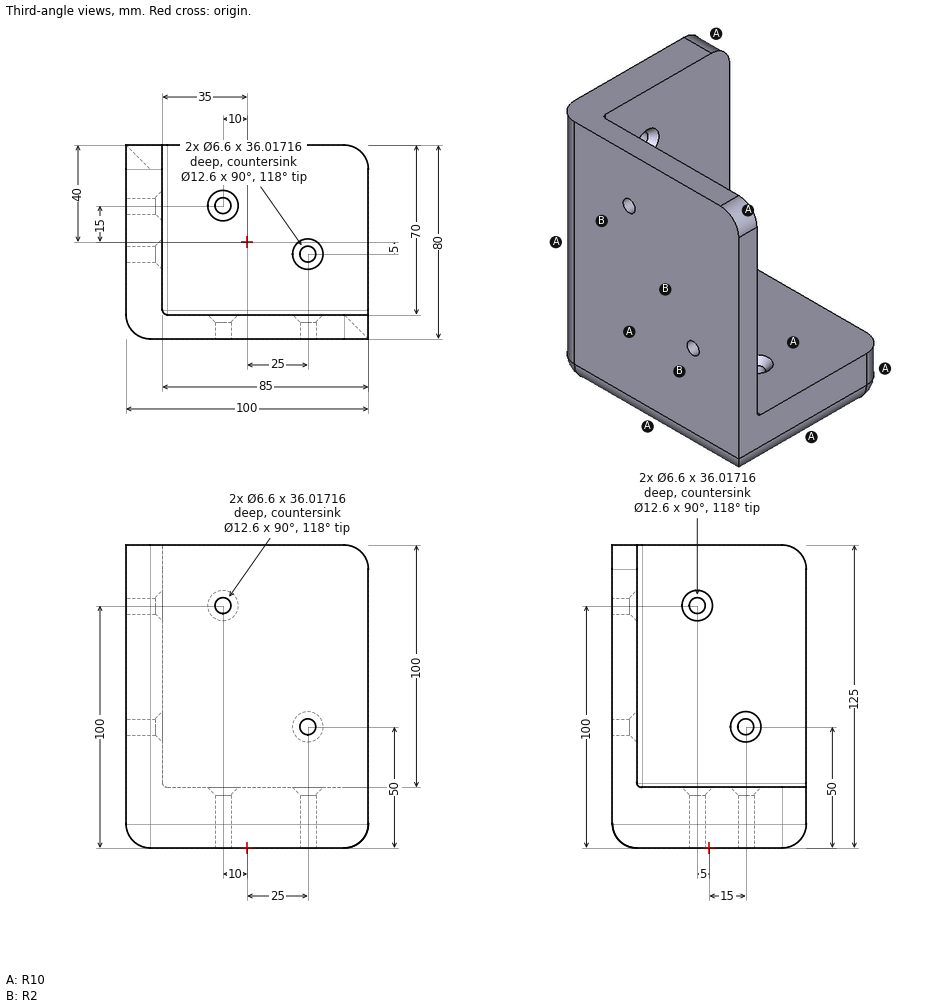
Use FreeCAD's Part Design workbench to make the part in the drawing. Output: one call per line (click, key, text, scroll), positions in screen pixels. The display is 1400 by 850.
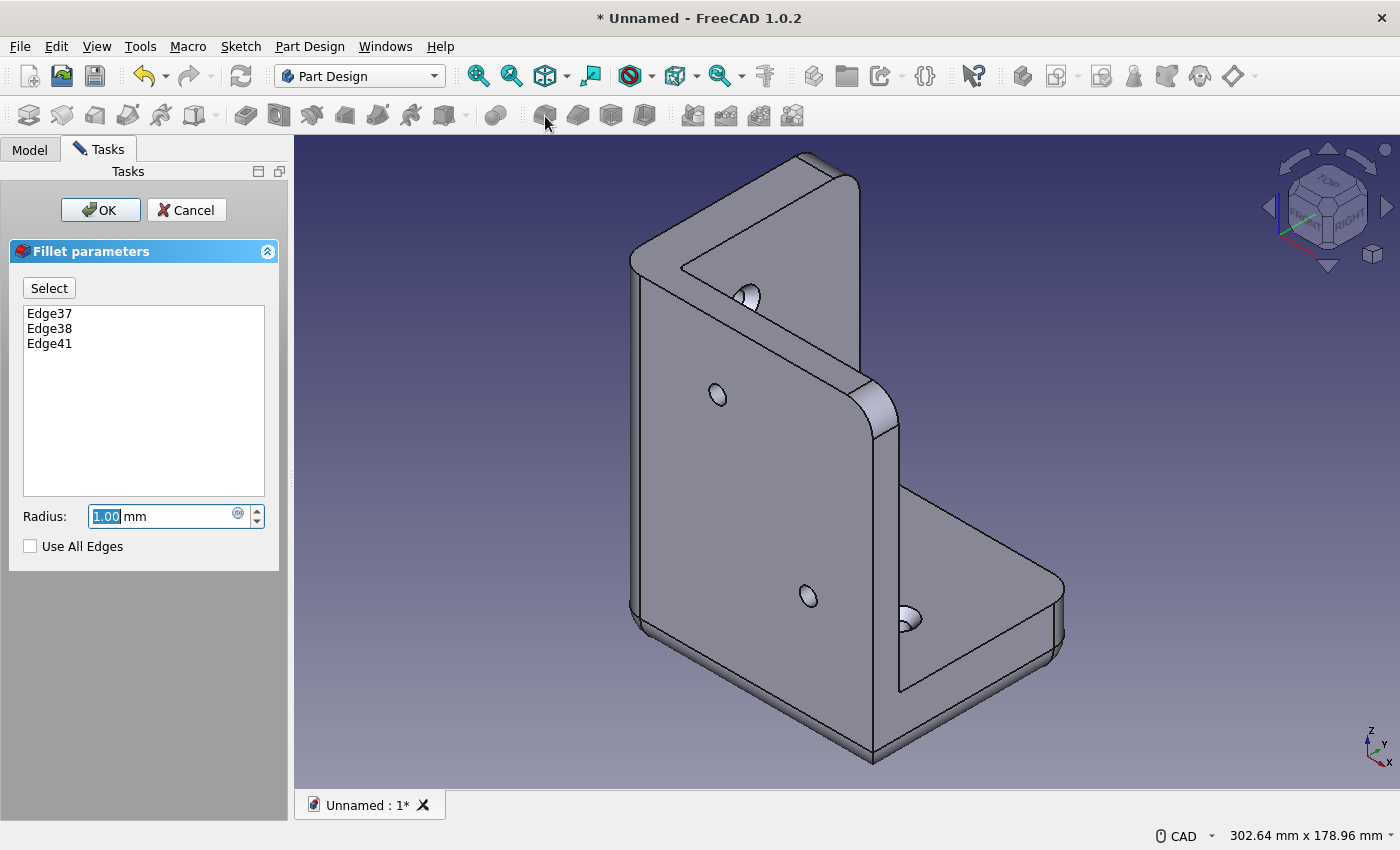
text(2)
key(Tab)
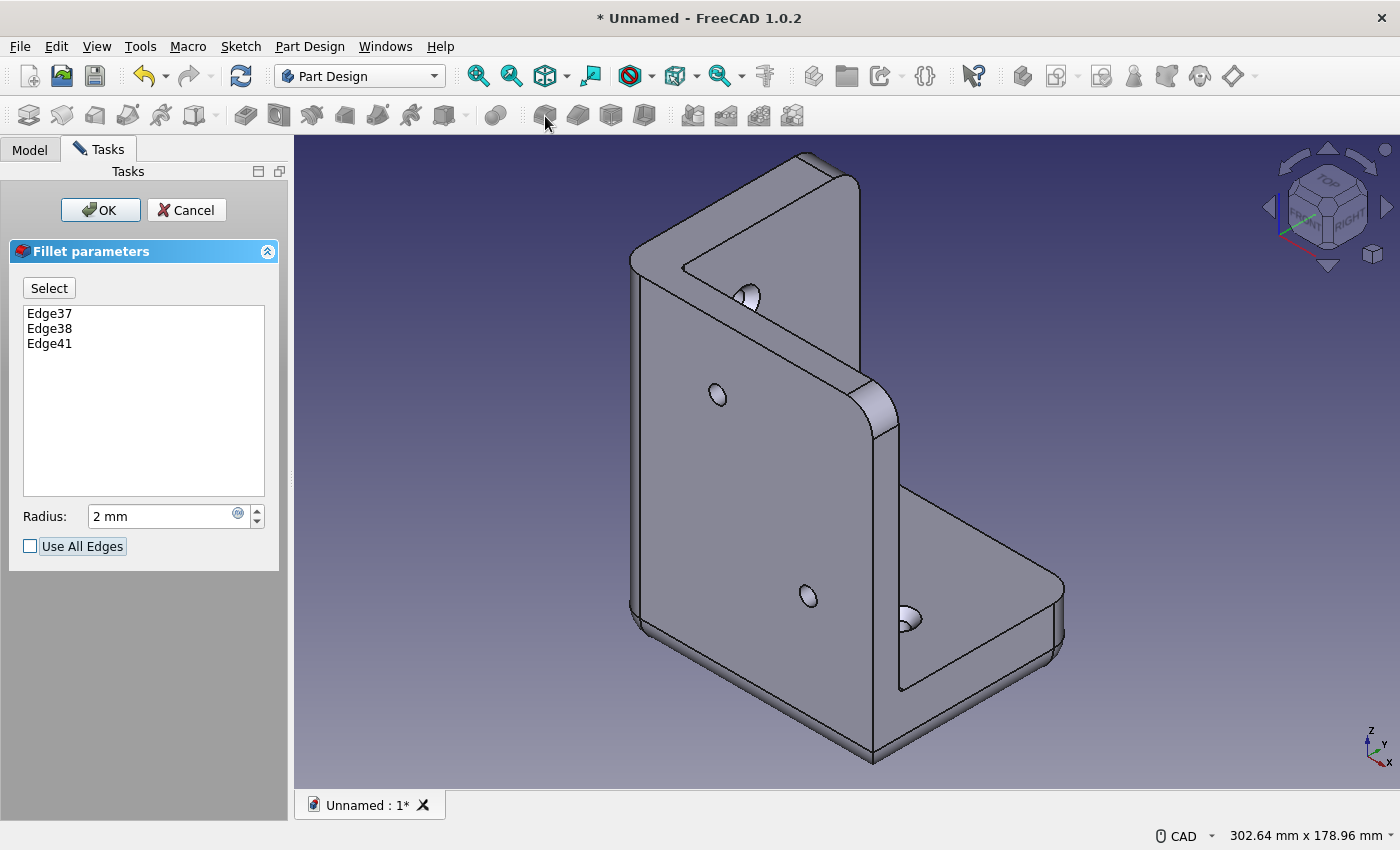
click(101, 210)